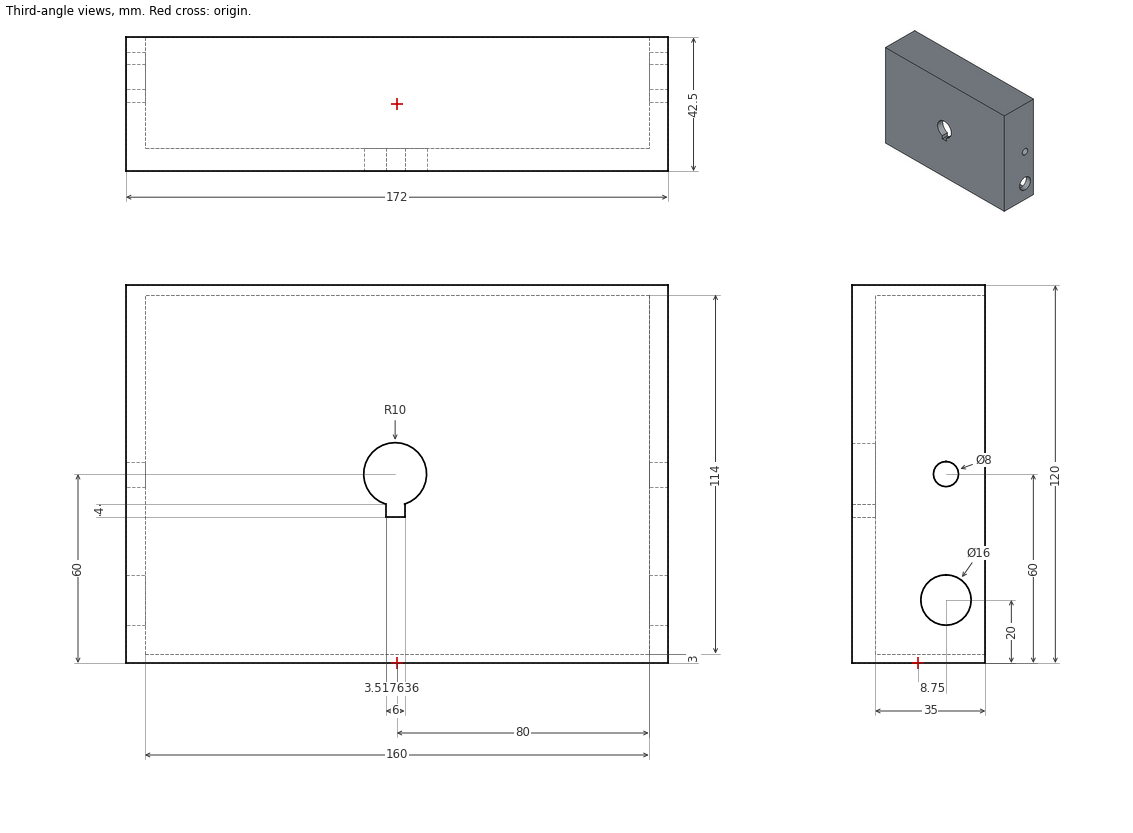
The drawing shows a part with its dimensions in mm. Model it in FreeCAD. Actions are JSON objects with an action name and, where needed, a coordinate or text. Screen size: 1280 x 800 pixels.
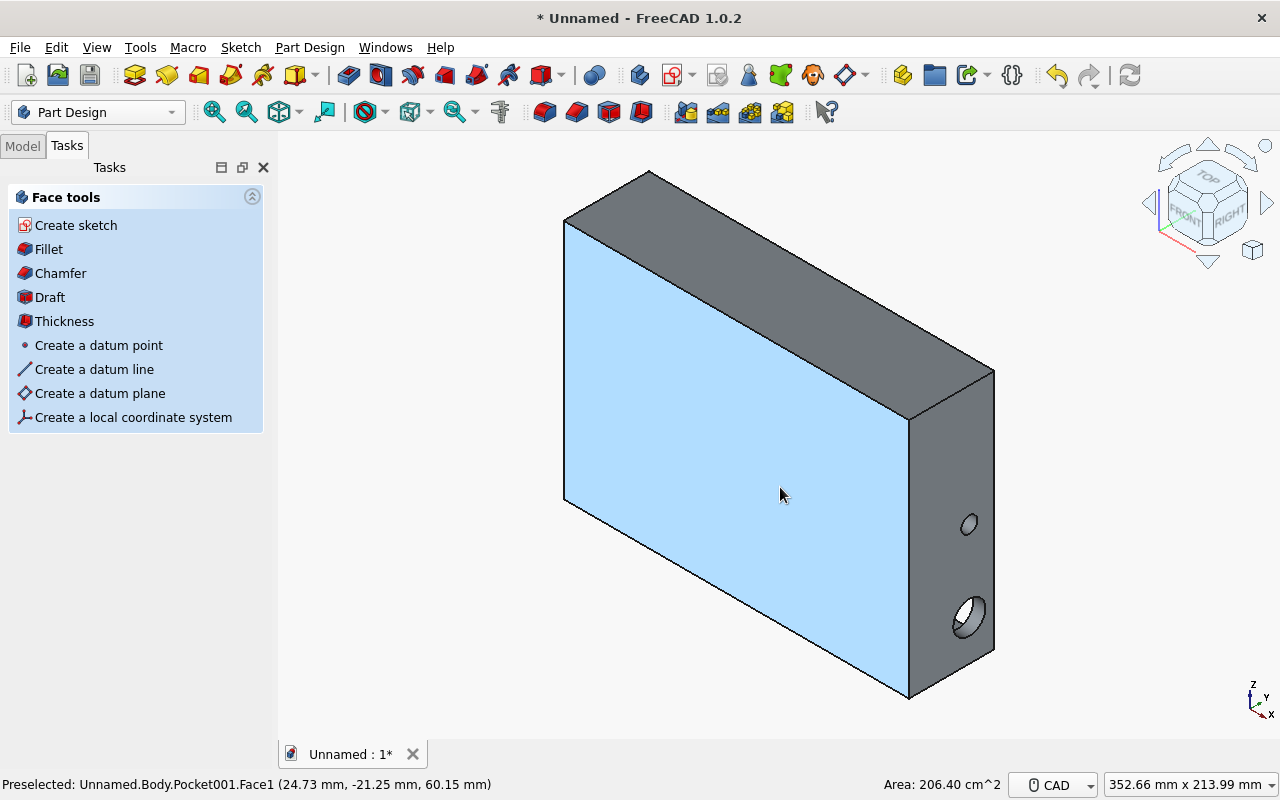
{"action": "left_click", "coordinate": [672, 76]}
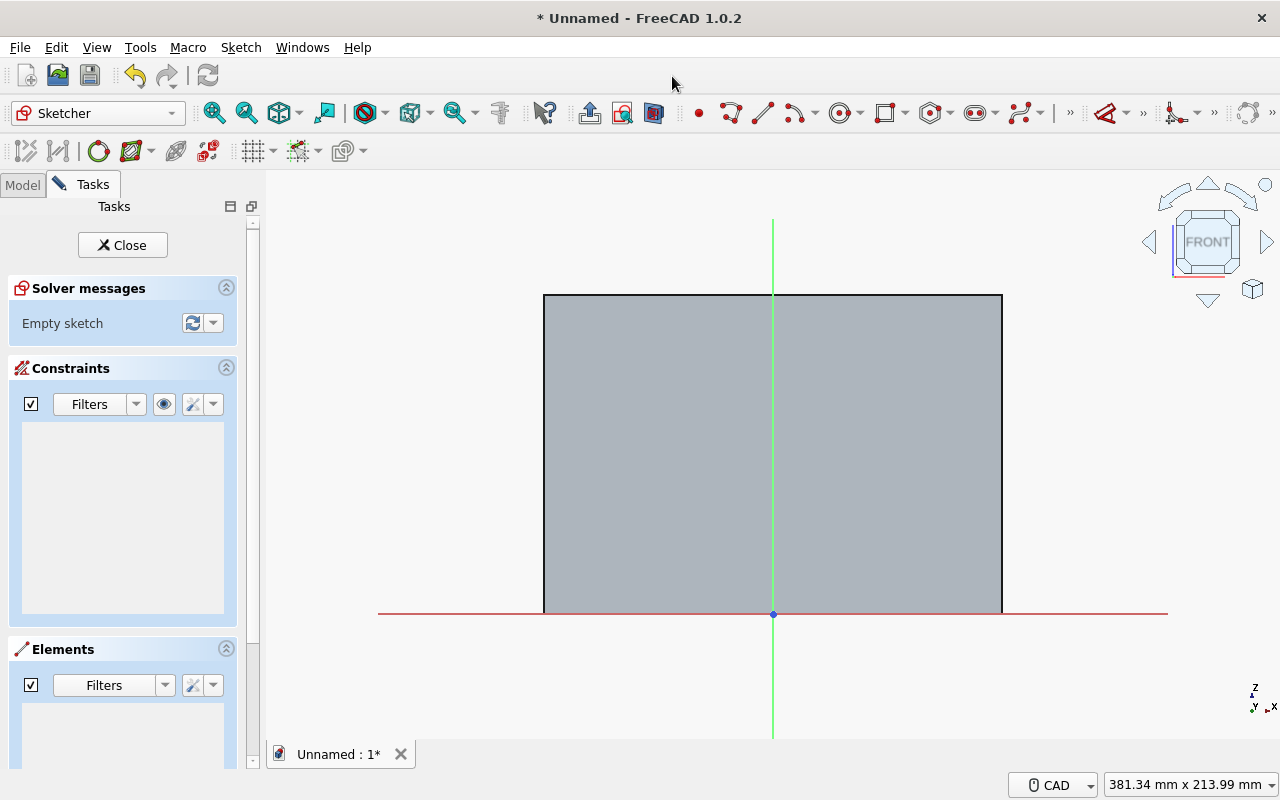
{"action": "scroll", "coordinate": [785, 460], "scroll_direction": "up", "scroll_amount": 9}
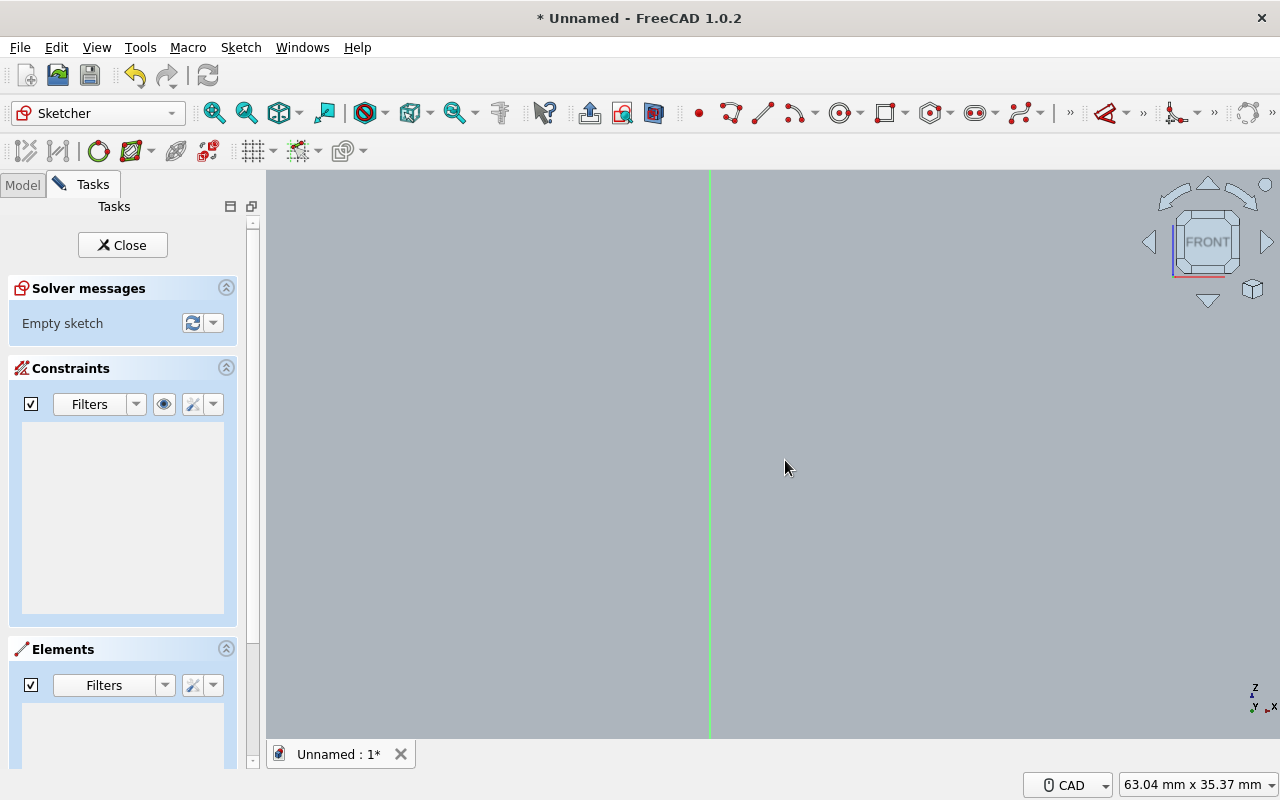
{"action": "left_click", "coordinate": [732, 114]}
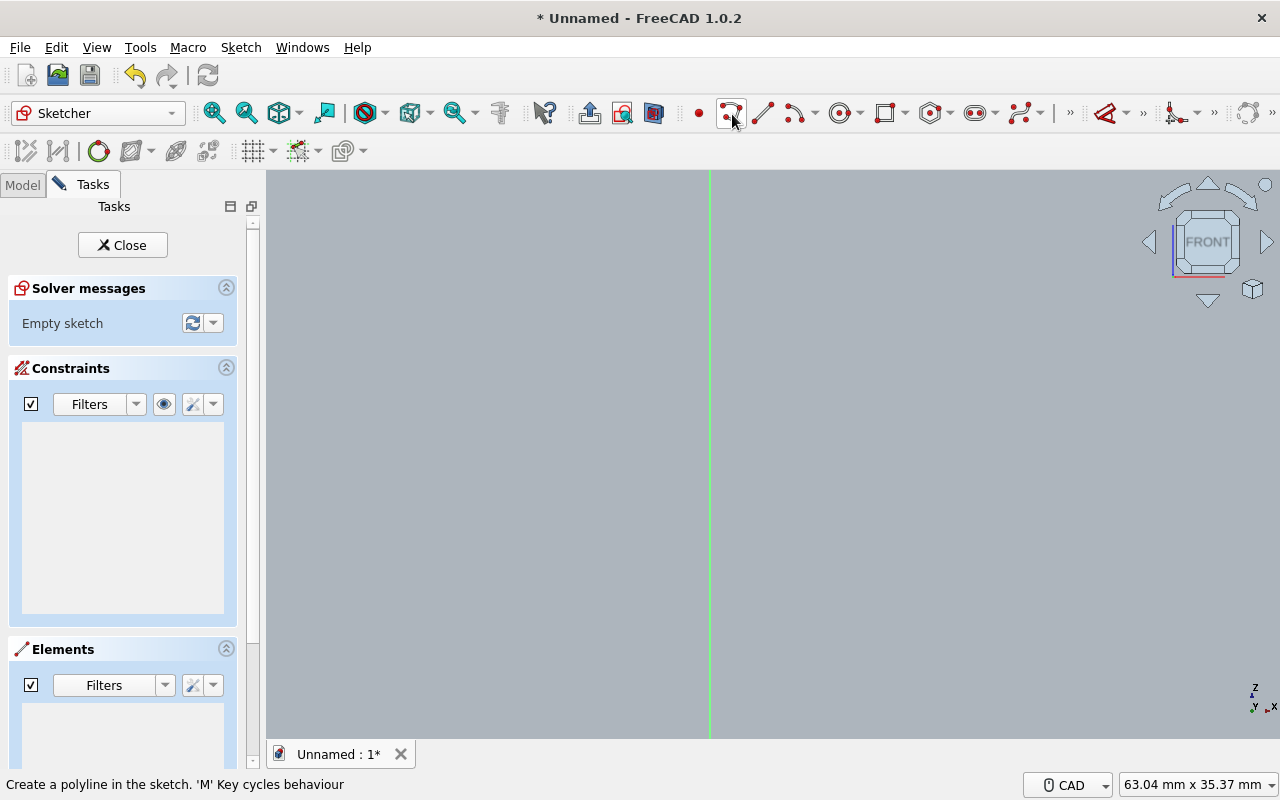
{"action": "left_click", "coordinate": [653, 578]}
{"action": "left_click", "coordinate": [653, 642]}
{"action": "left_click", "coordinate": [750, 642]}
{"action": "left_click", "coordinate": [750, 578]}
{"action": "right_click", "coordinate": [750, 578]}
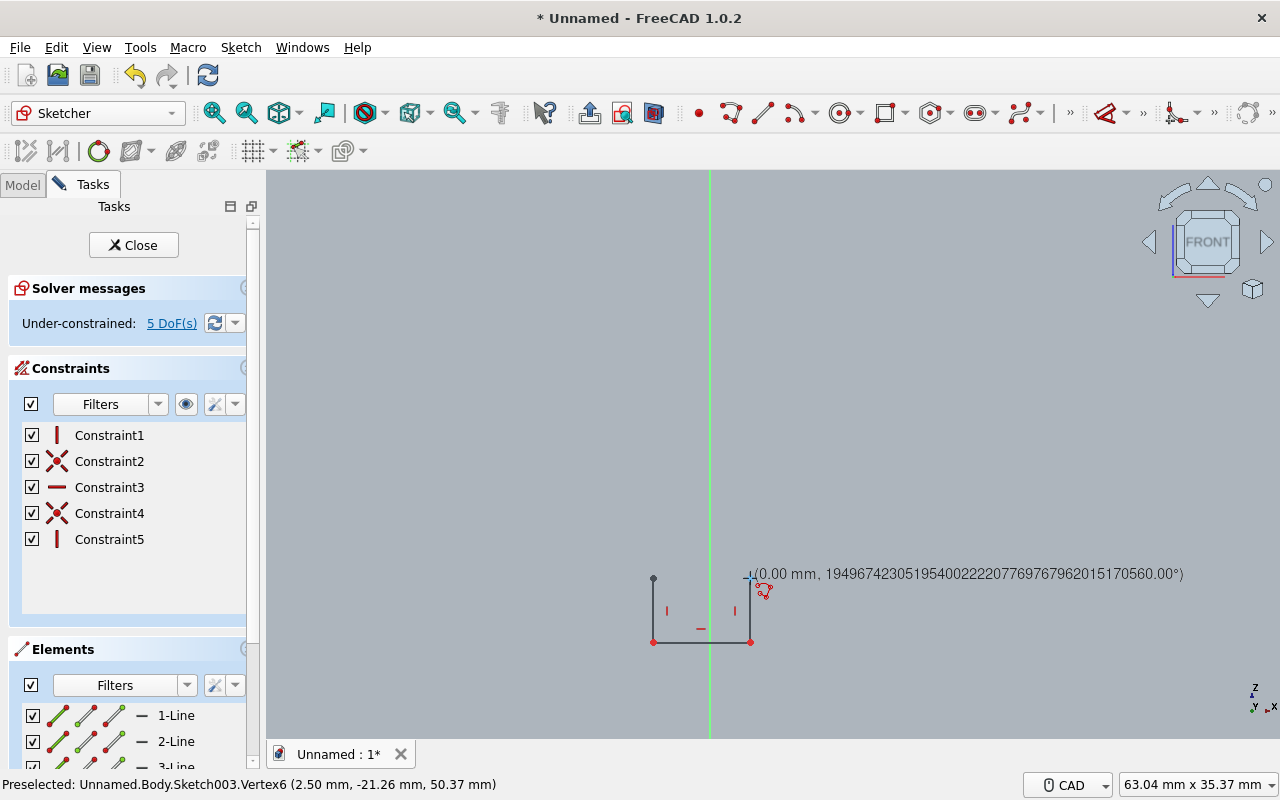
{"action": "key", "text": "g 3 a"}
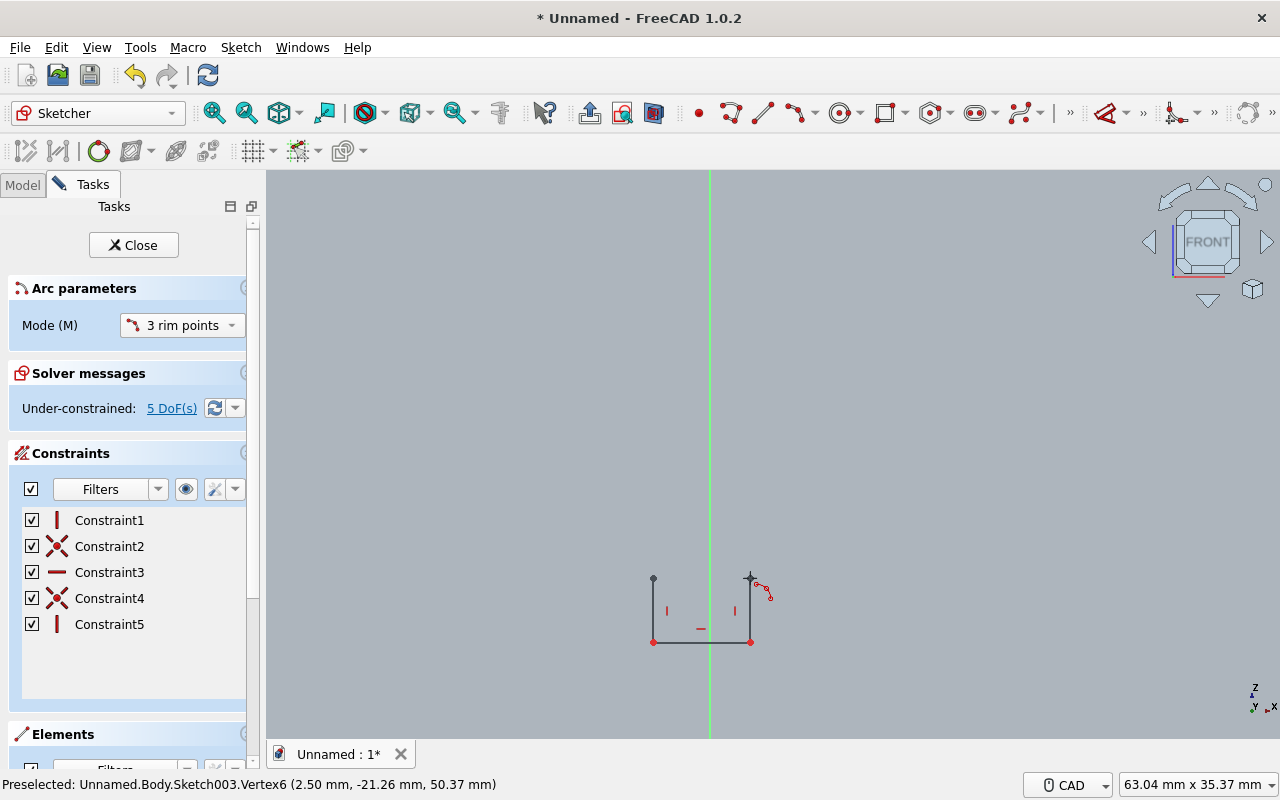
{"action": "left_click", "coordinate": [750, 579]}
{"action": "left_click", "coordinate": [653, 579]}
{"action": "left_click", "coordinate": [788, 288]}
{"action": "key", "text": "Escape"}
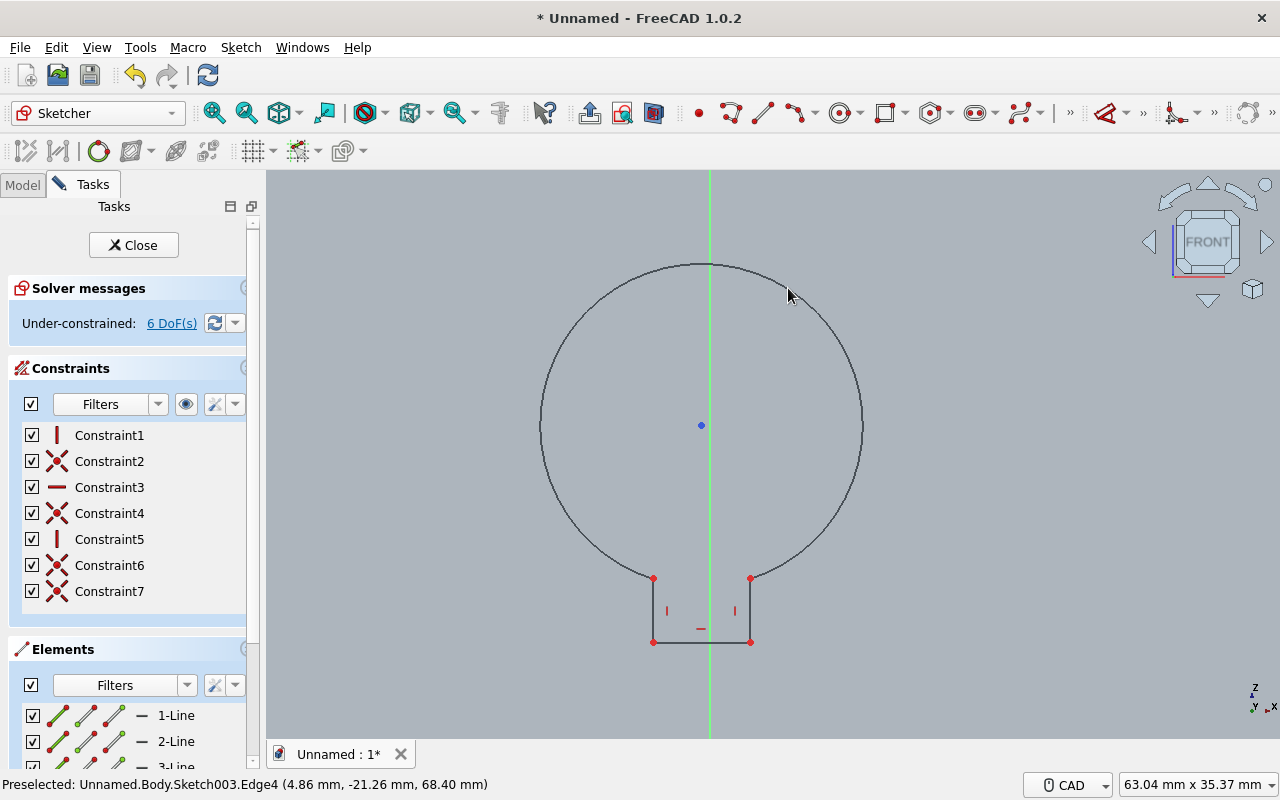
{"action": "left_click", "coordinate": [1106, 114]}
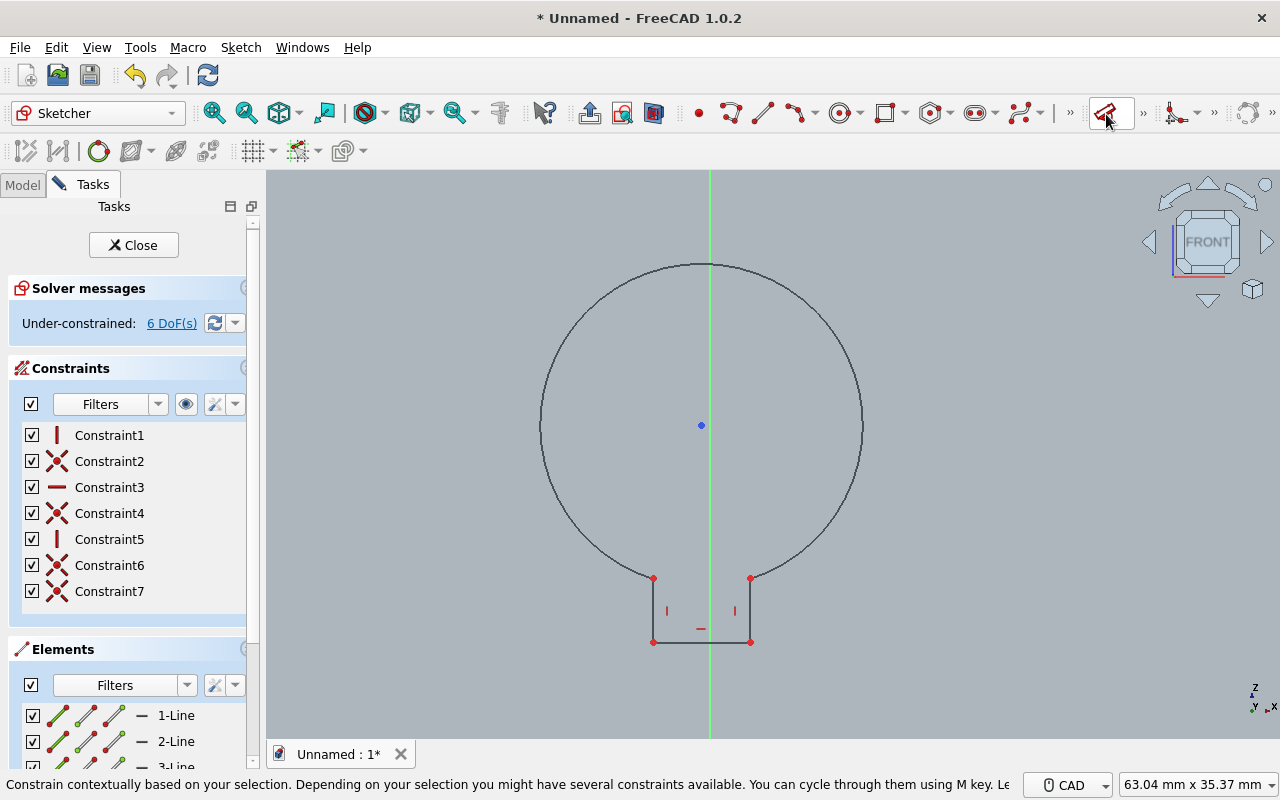
{"action": "left_click", "coordinate": [848, 357]}
{"action": "left_click", "coordinate": [877, 344]}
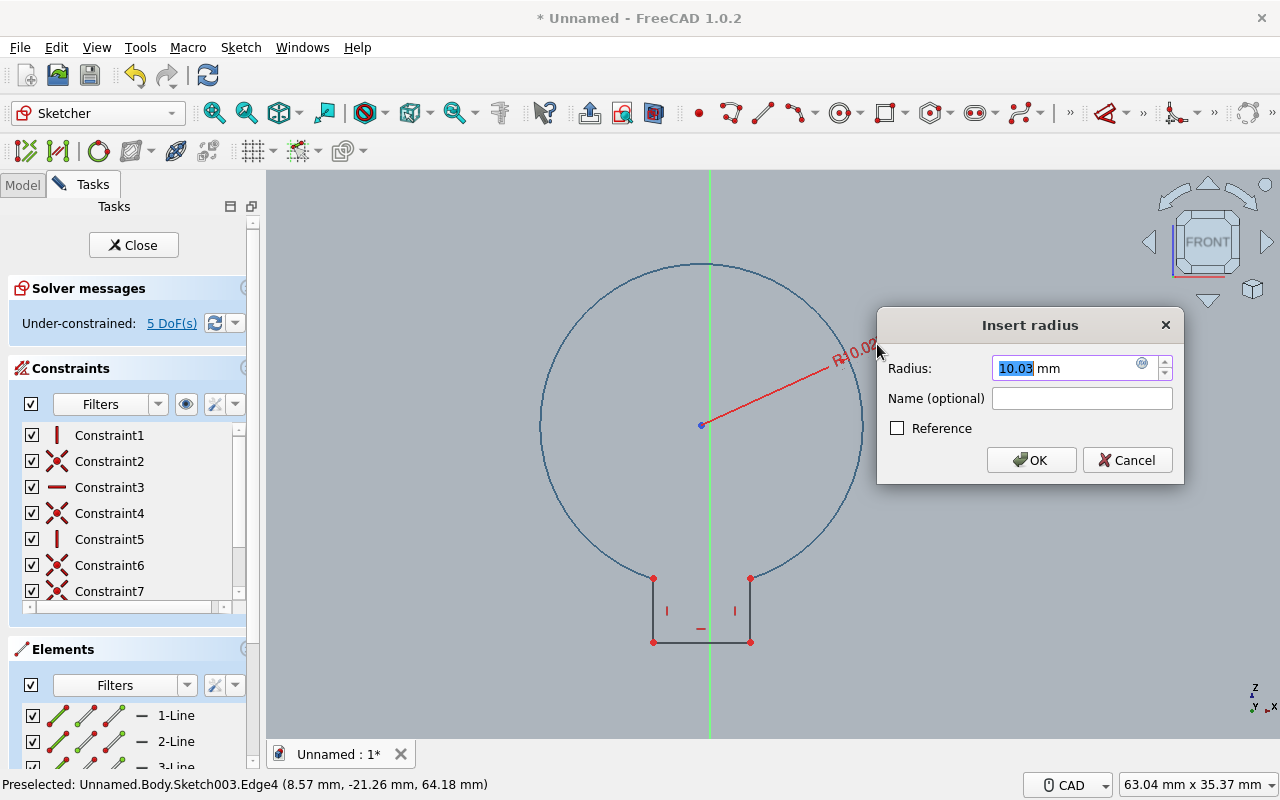
{"action": "type", "text": "10"}
{"action": "key", "text": "Return"}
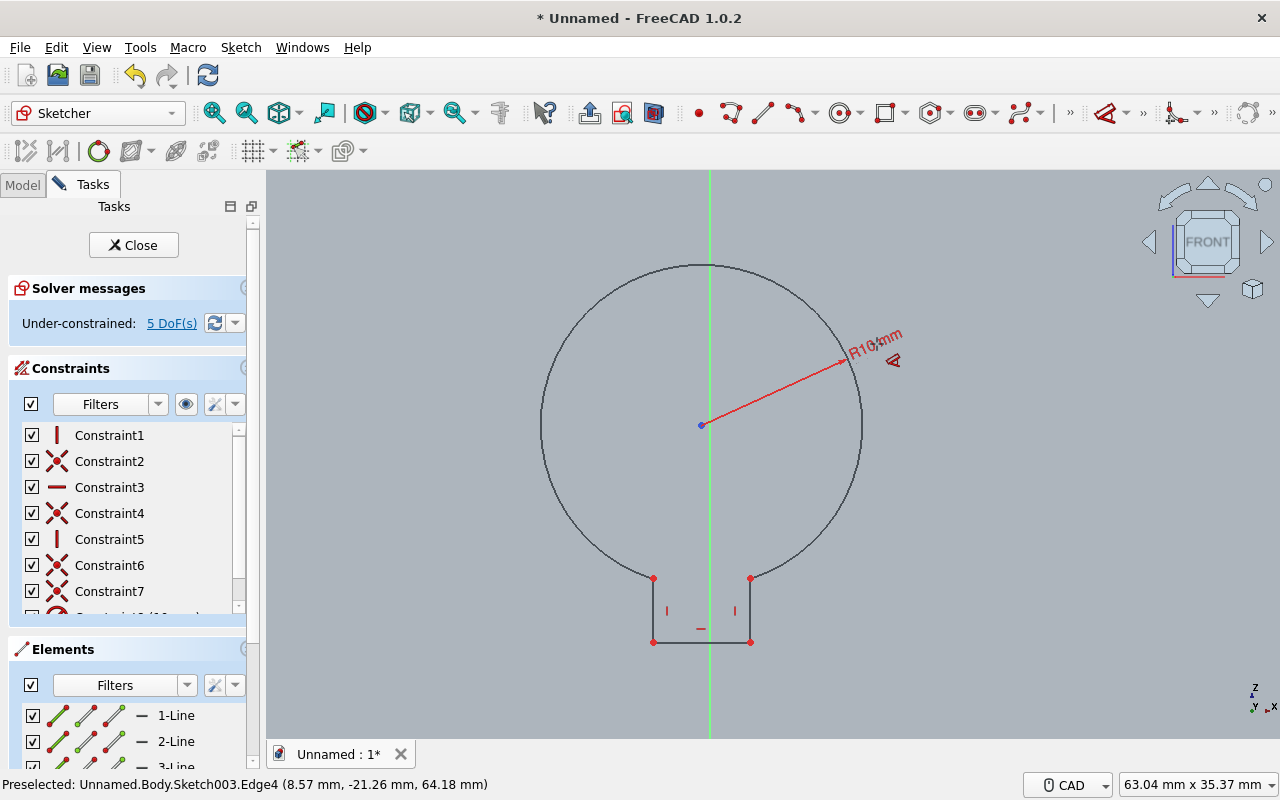
{"action": "left_click", "coordinate": [653, 598]}
{"action": "left_click", "coordinate": [619, 611]}